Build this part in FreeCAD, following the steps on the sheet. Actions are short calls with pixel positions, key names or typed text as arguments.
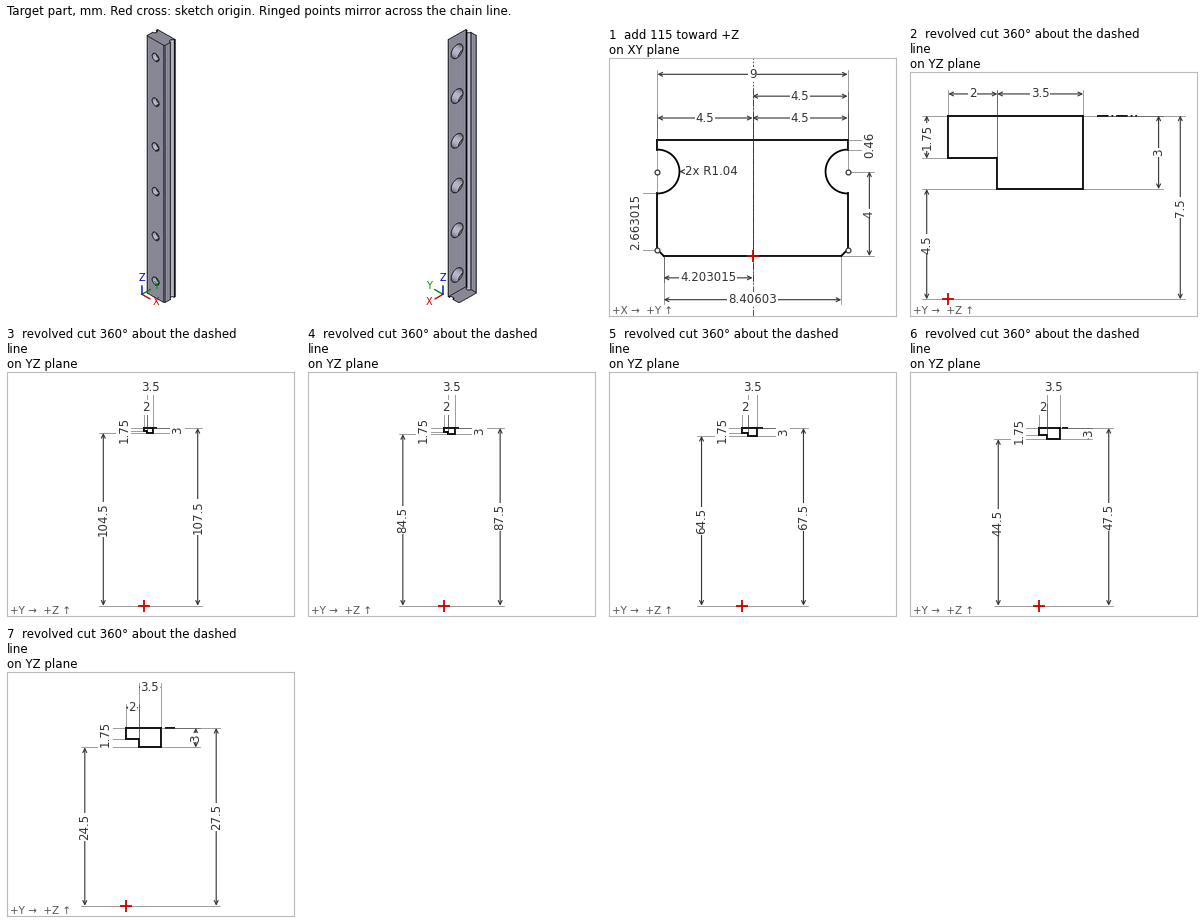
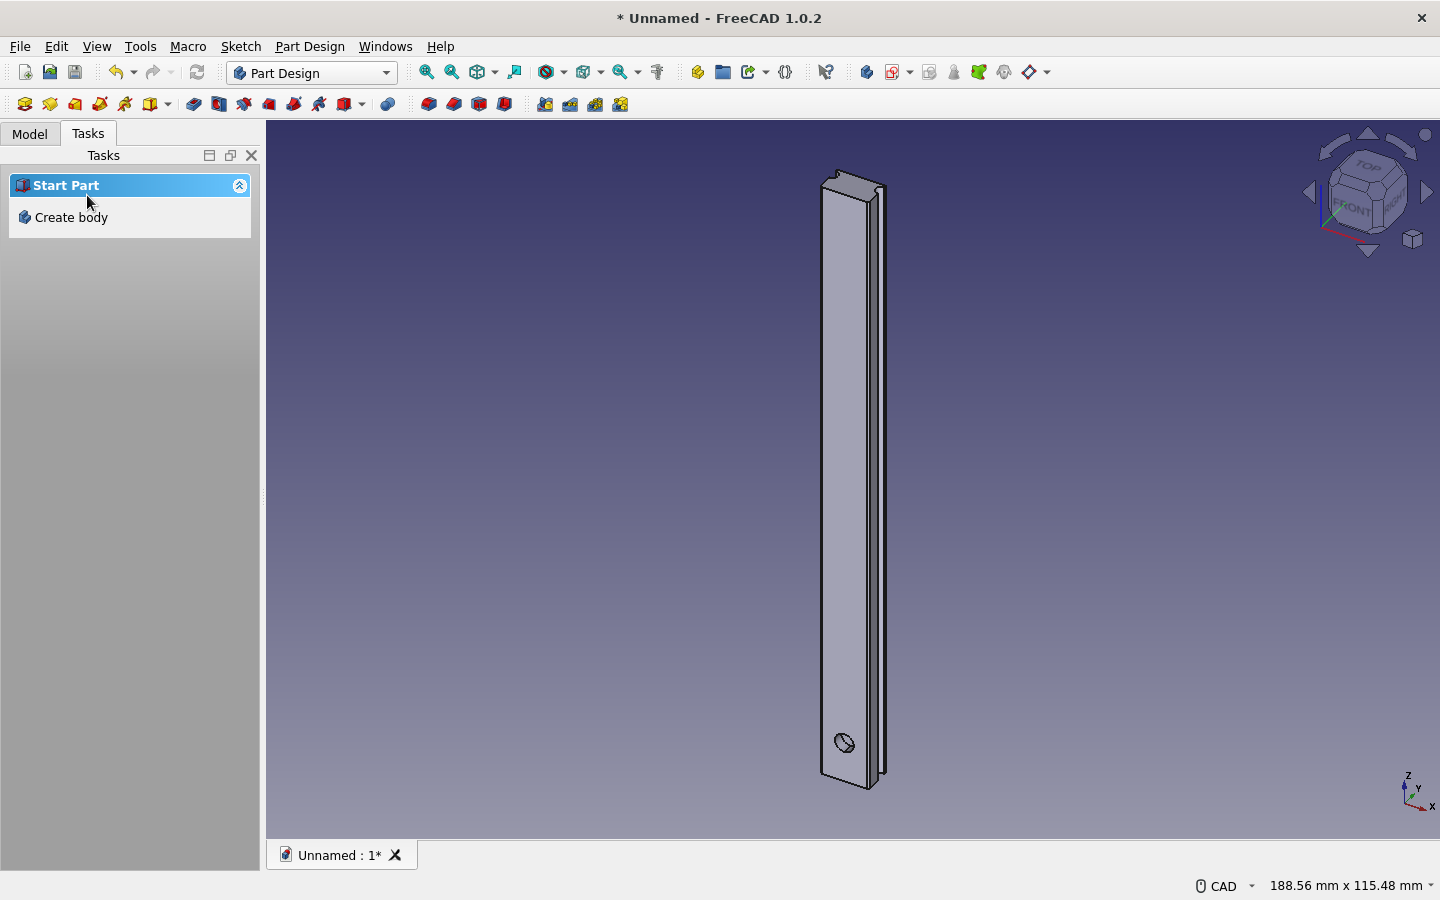
click(892, 72)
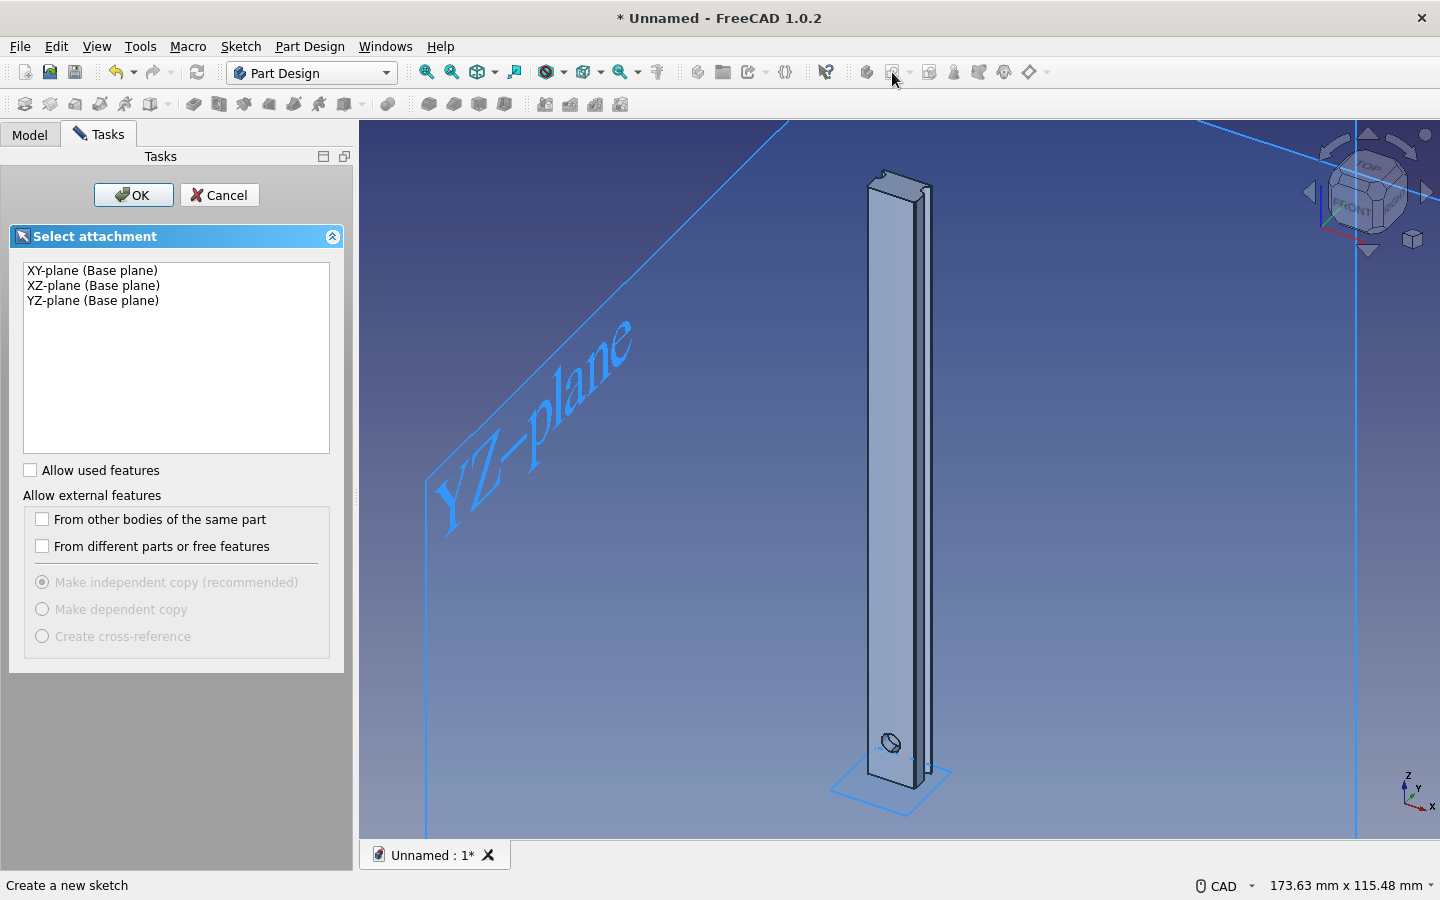
click(84, 300)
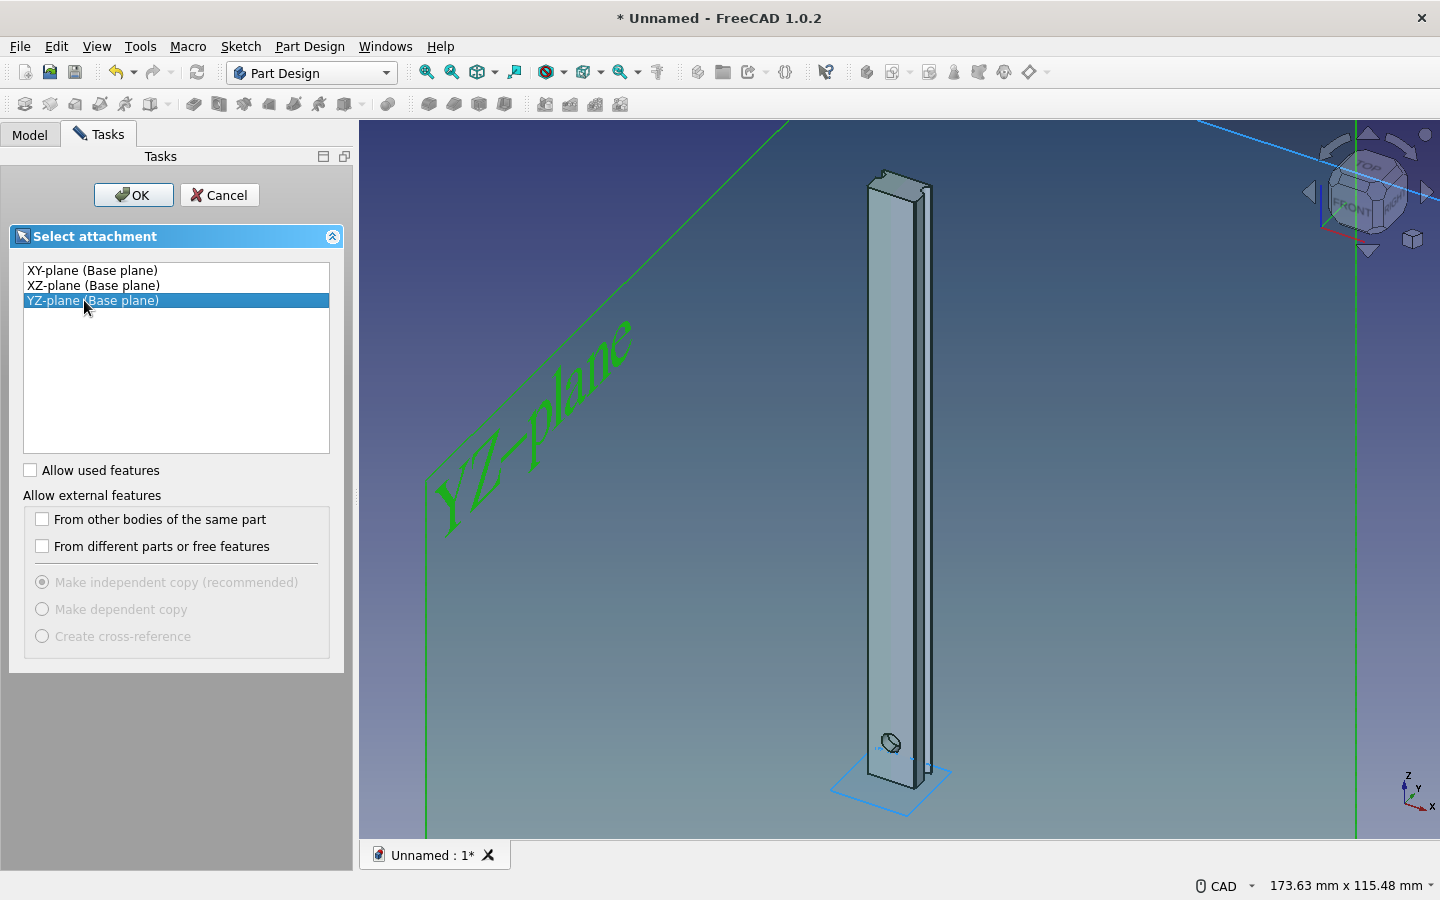
click(134, 195)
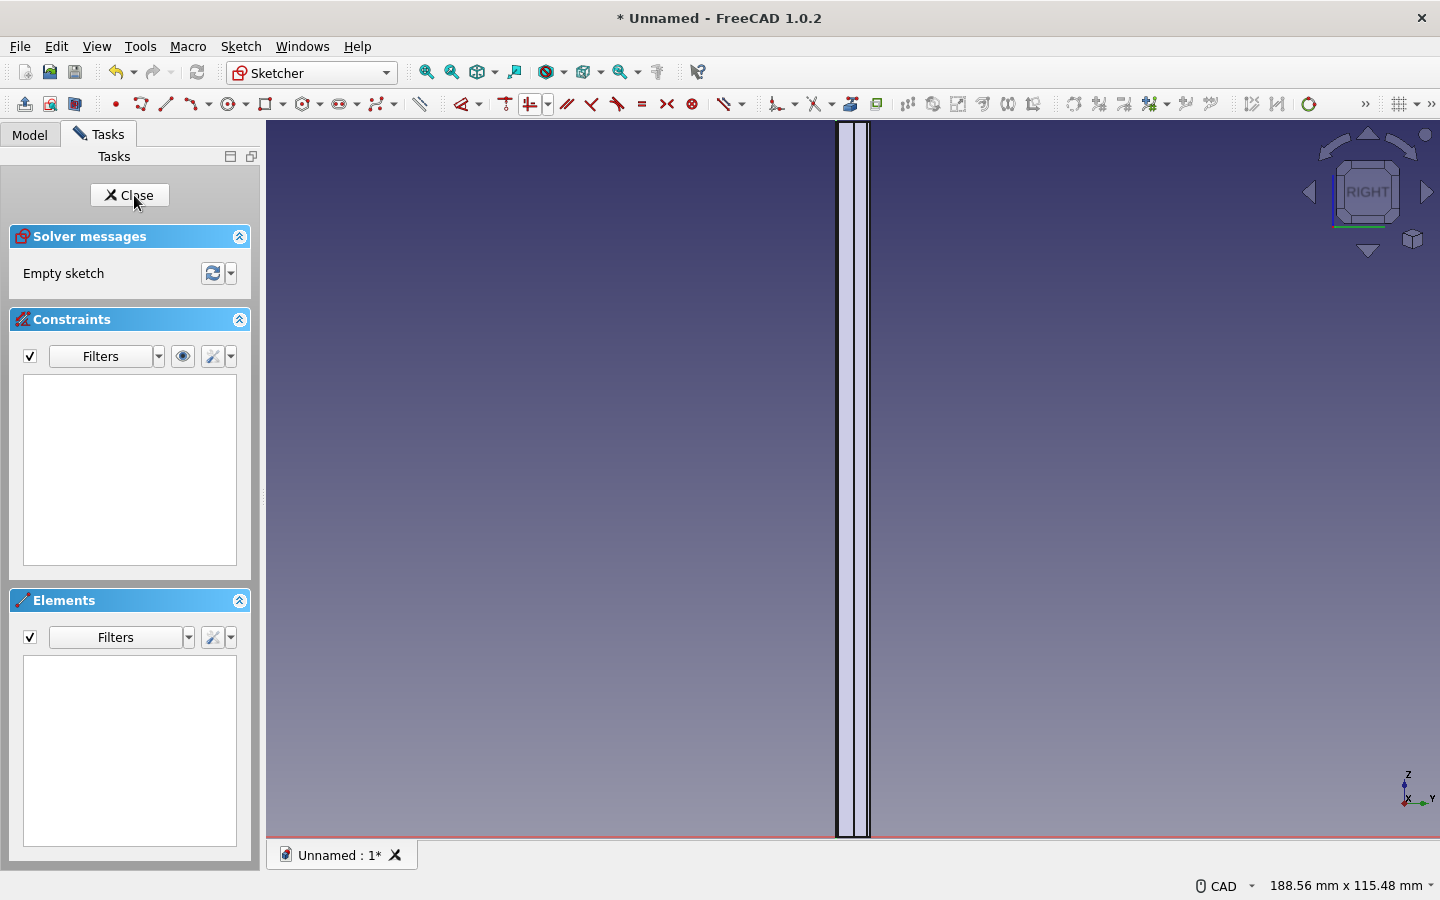
click(75, 104)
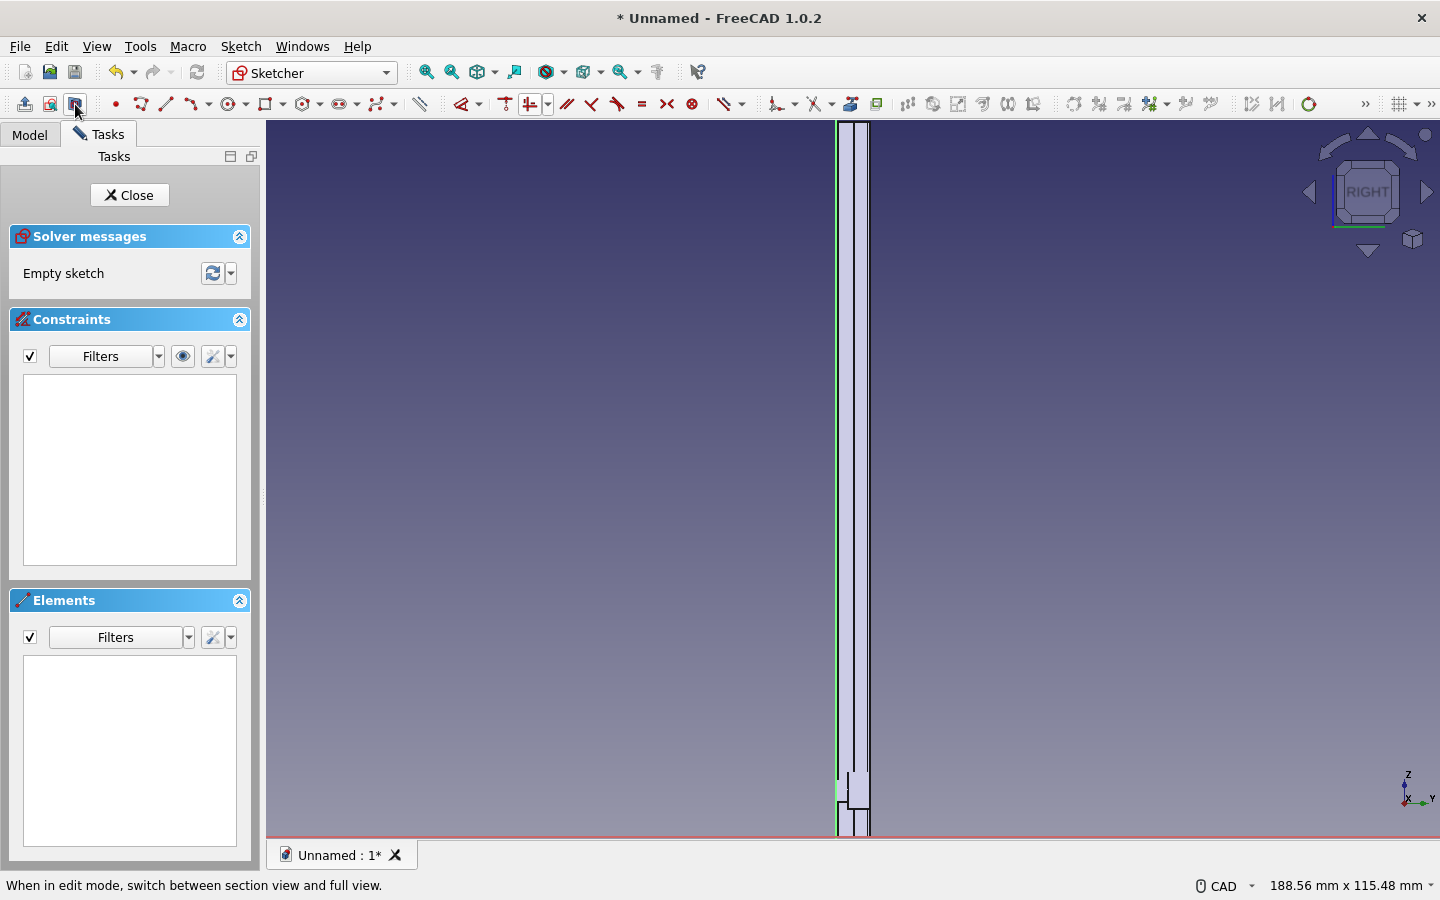
scroll(866, 153, up, 13)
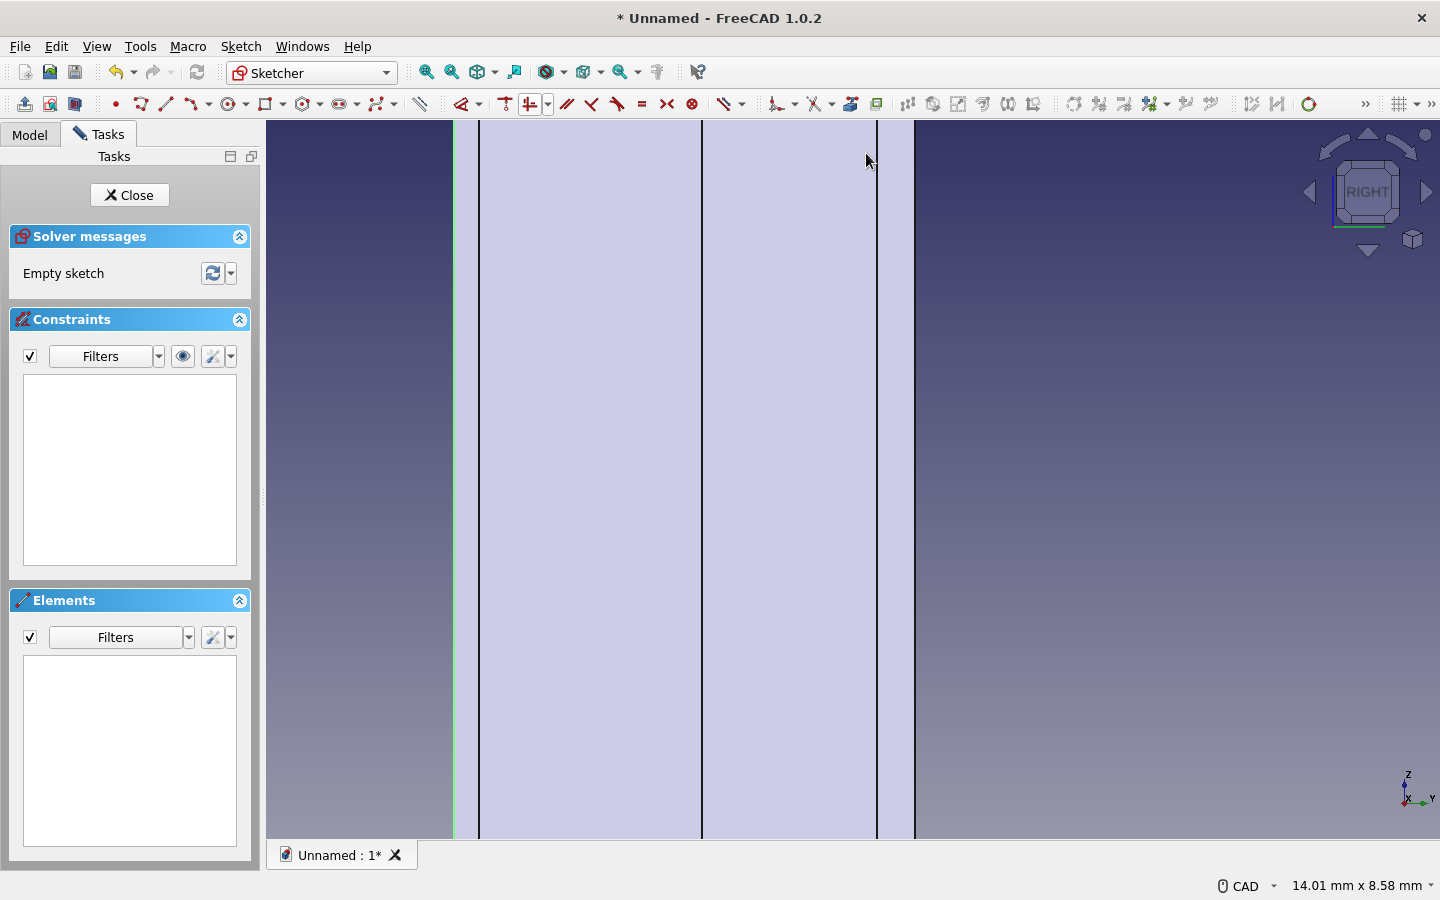
key(g)
key(m)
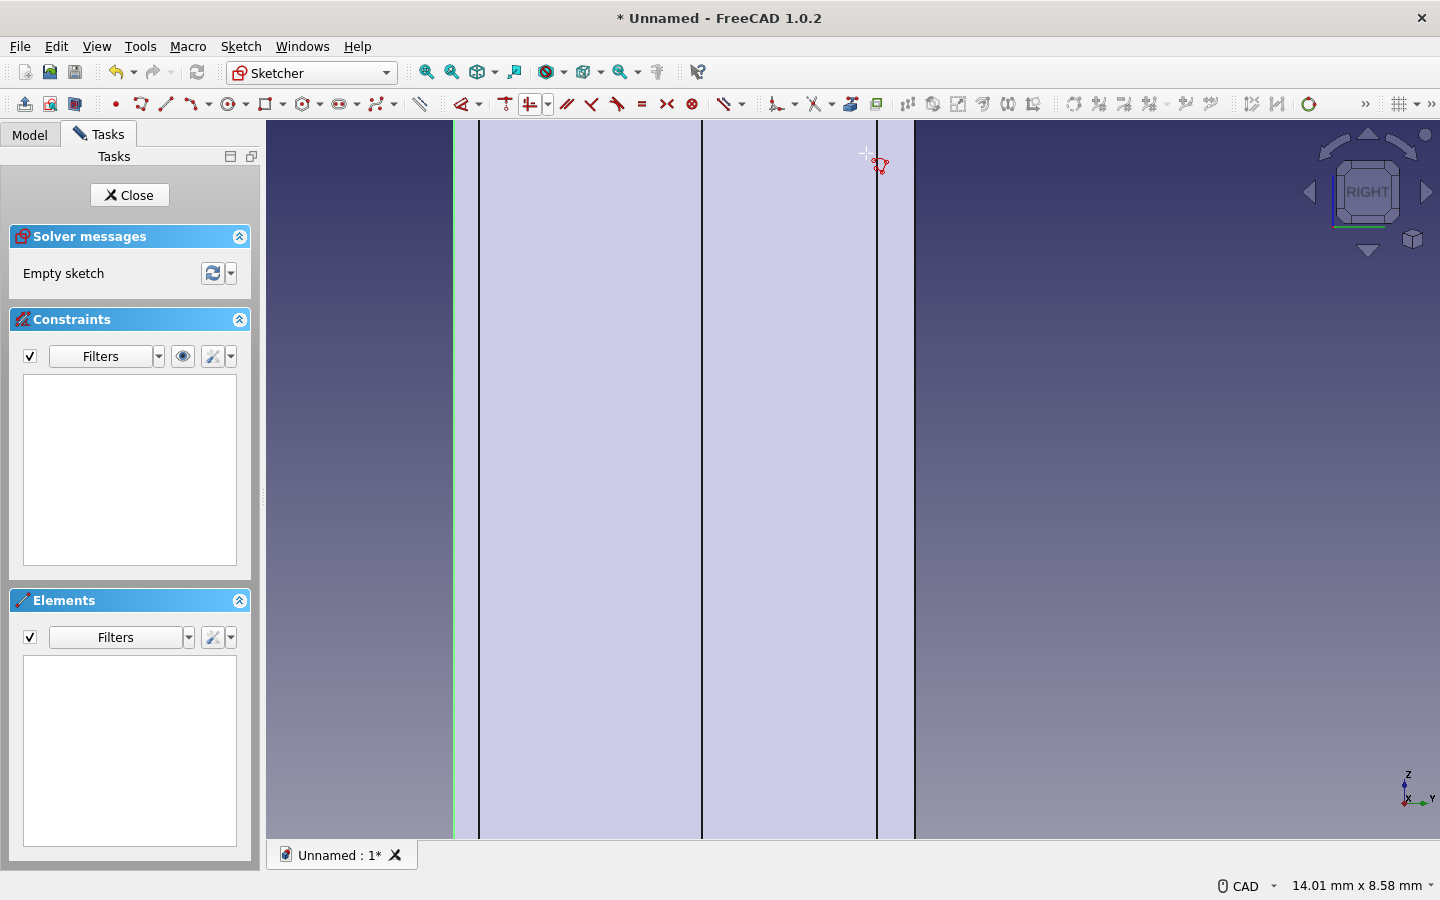
click(622, 609)
click(915, 609)
click(915, 357)
click(454, 357)
click(463, 504)
click(622, 504)
click(622, 610)